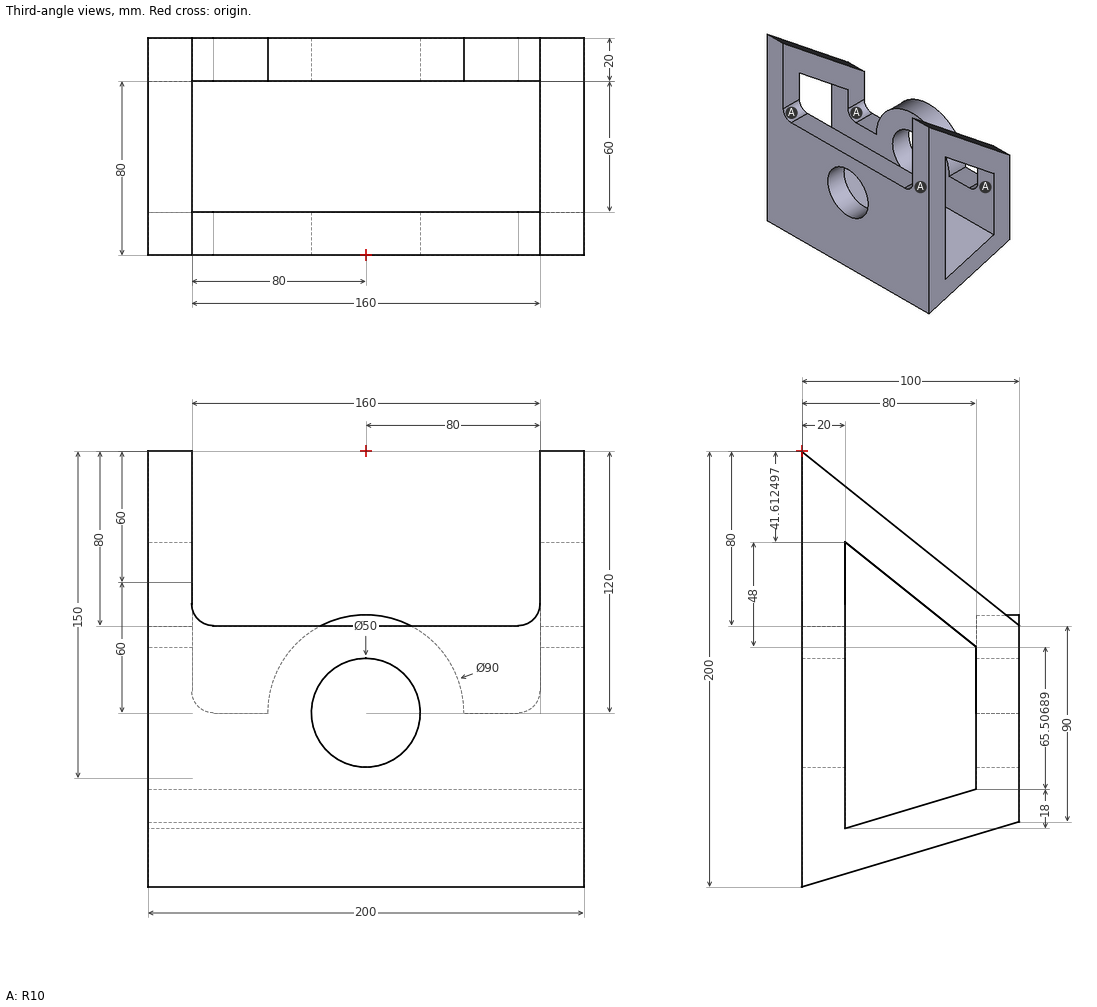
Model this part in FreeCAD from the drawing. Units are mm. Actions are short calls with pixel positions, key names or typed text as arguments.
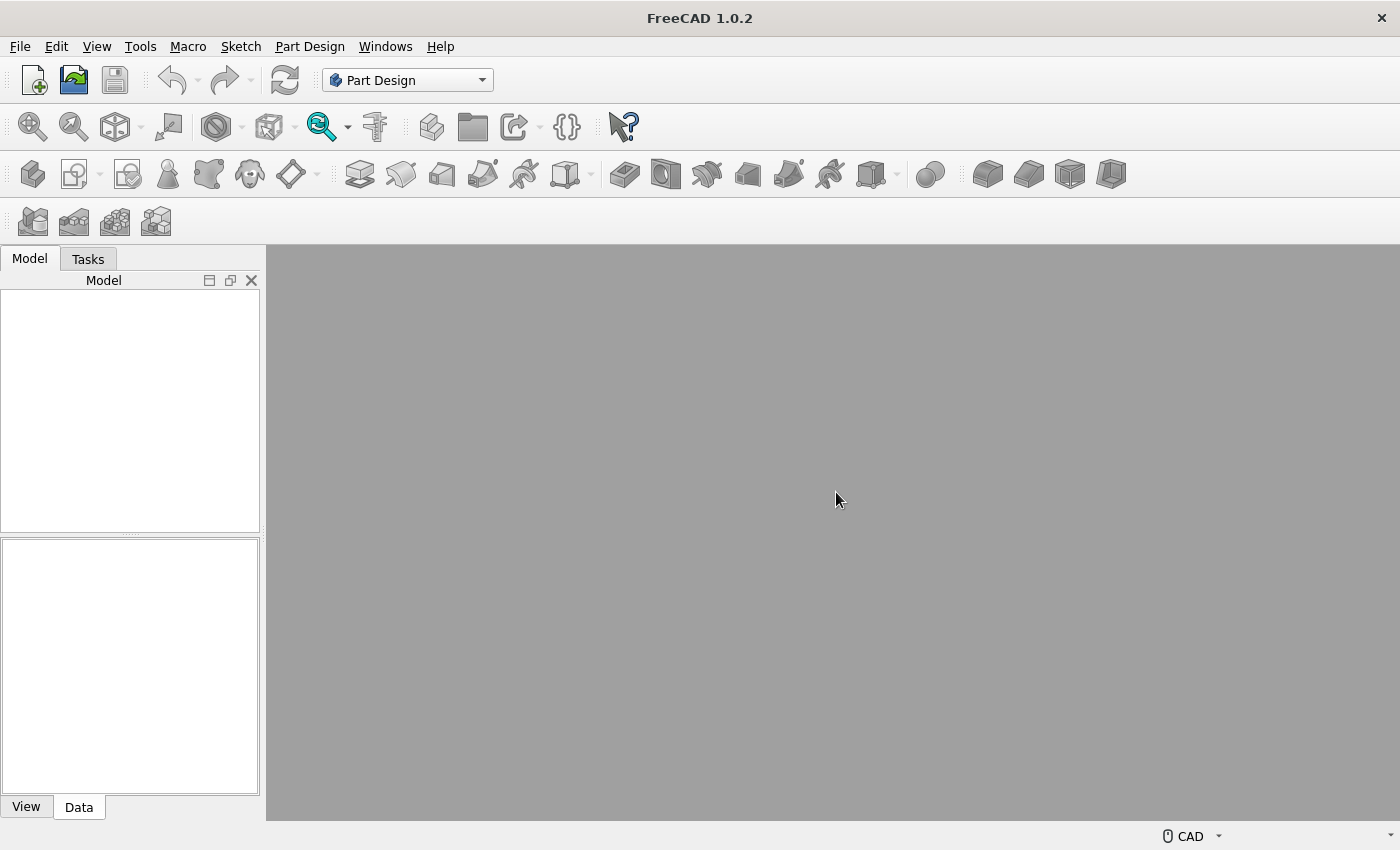
click(33, 80)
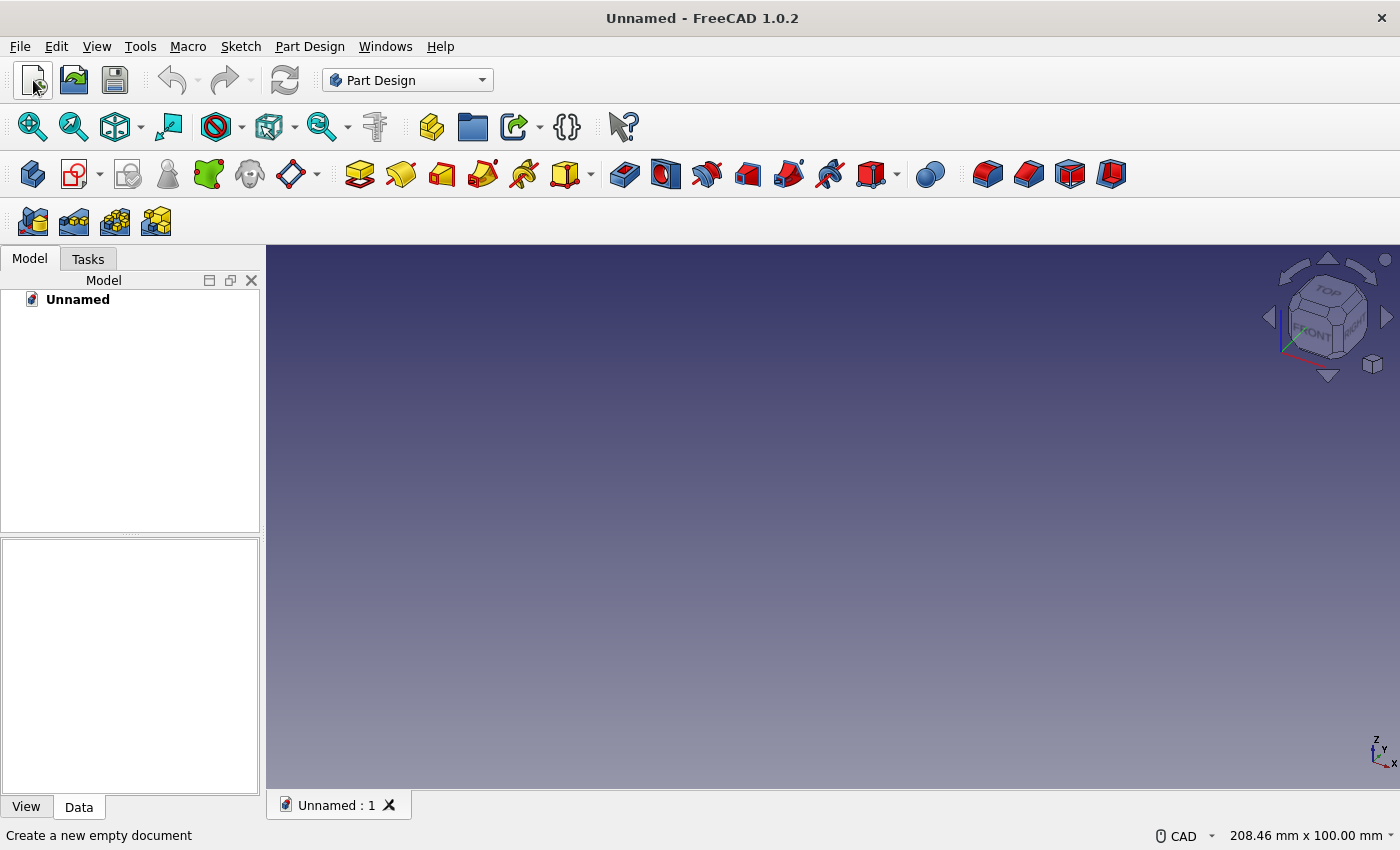
click(74, 174)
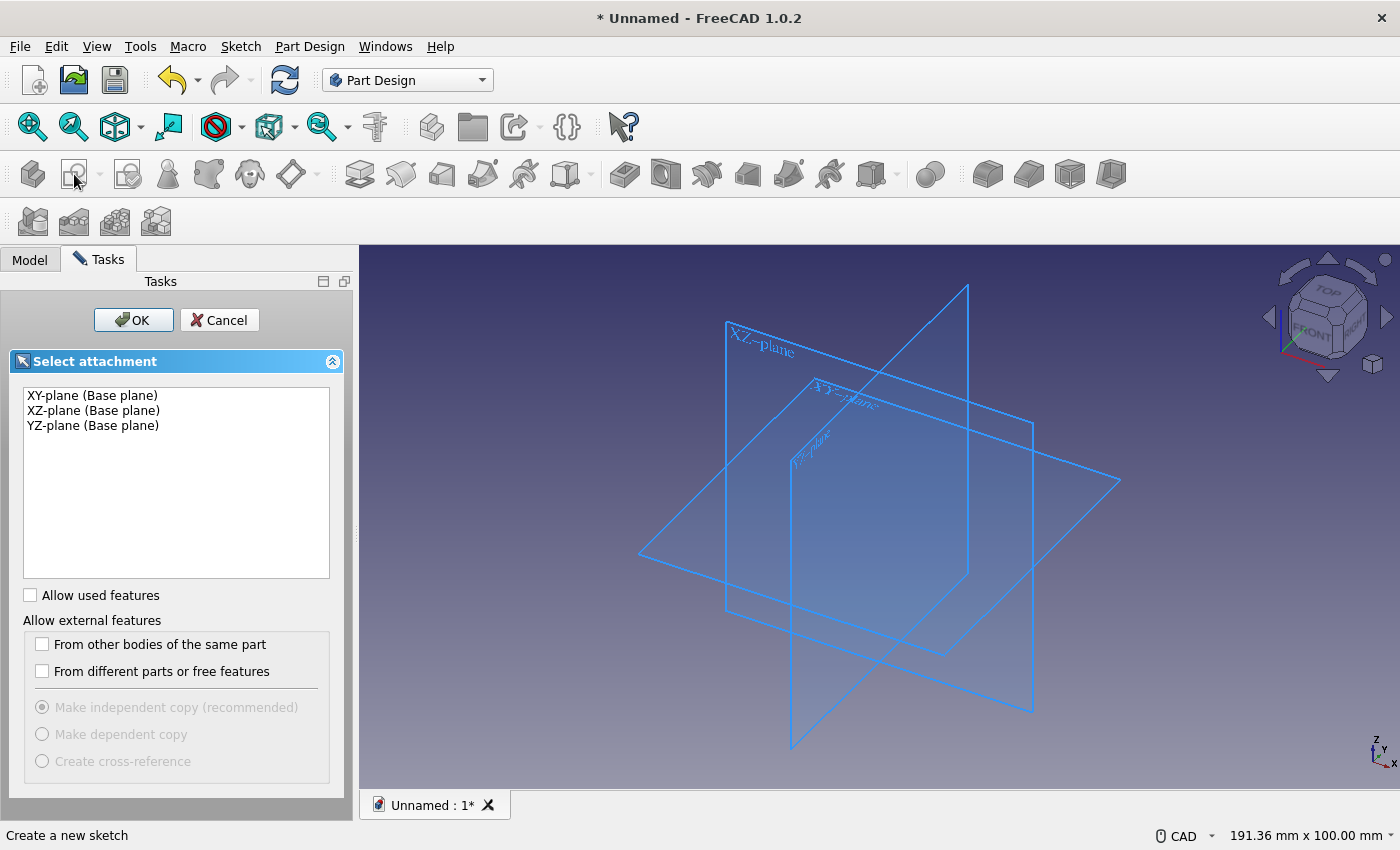
click(84, 426)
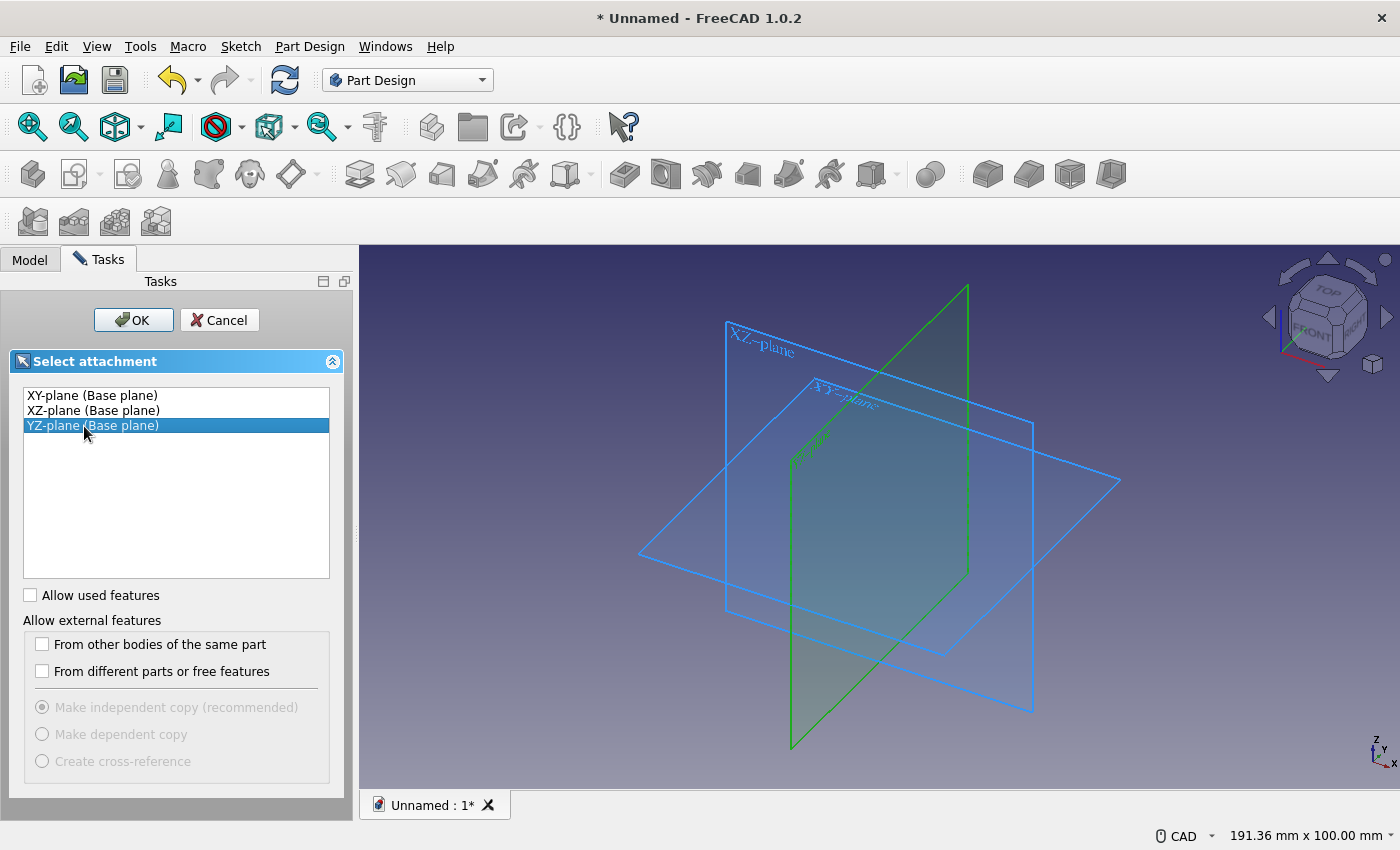
click(134, 320)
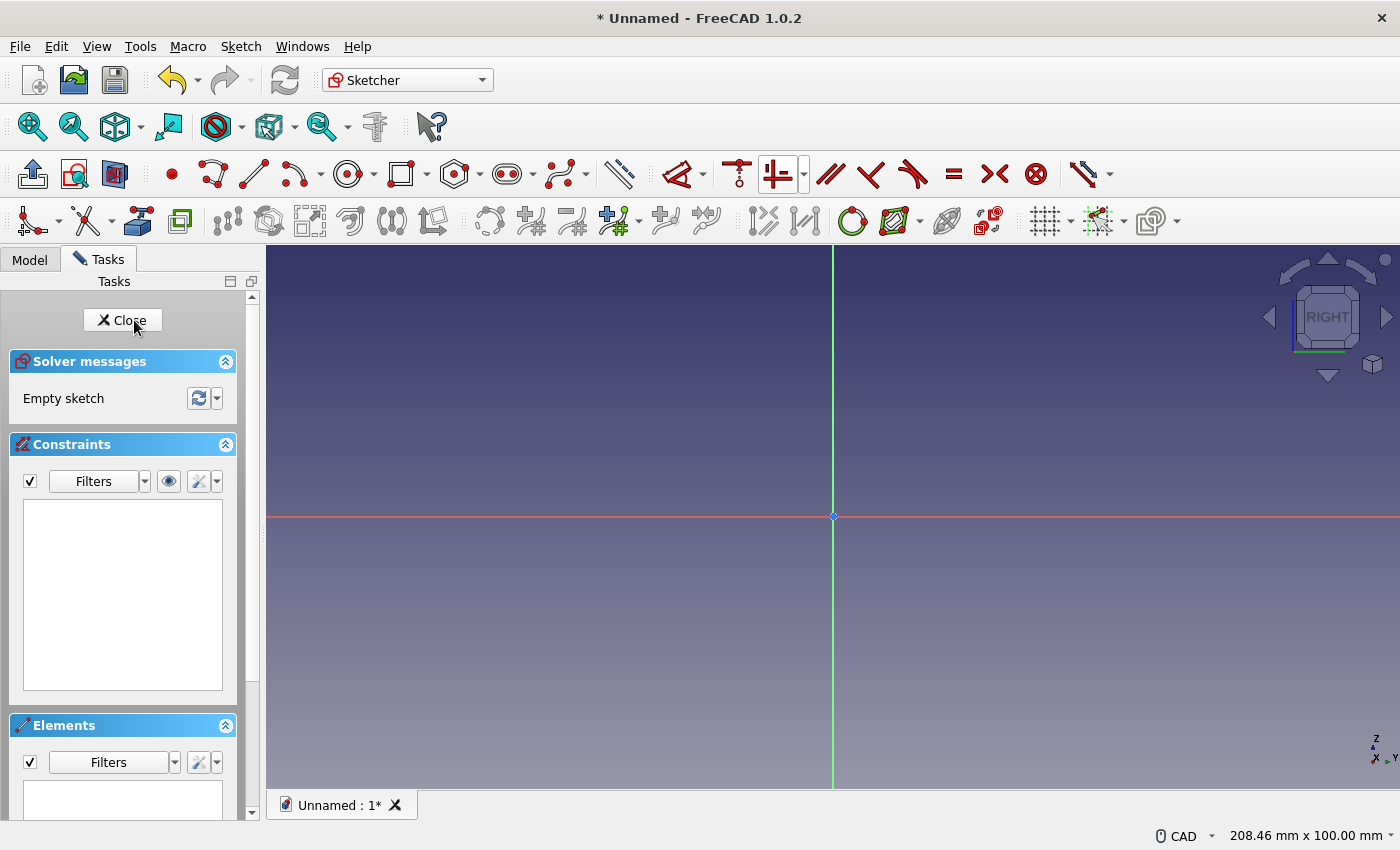
scroll(618, 283, down, 6)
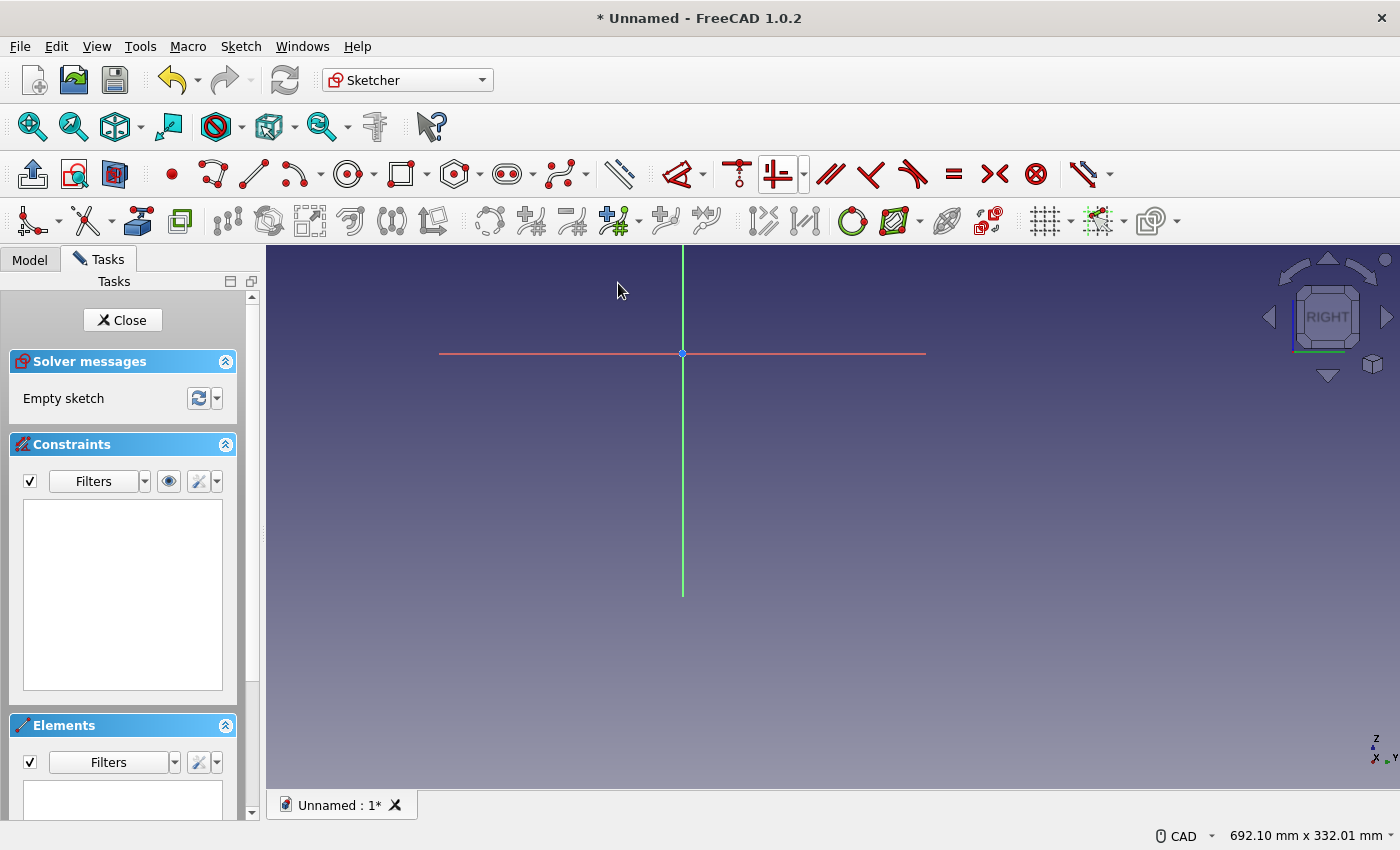
click(213, 174)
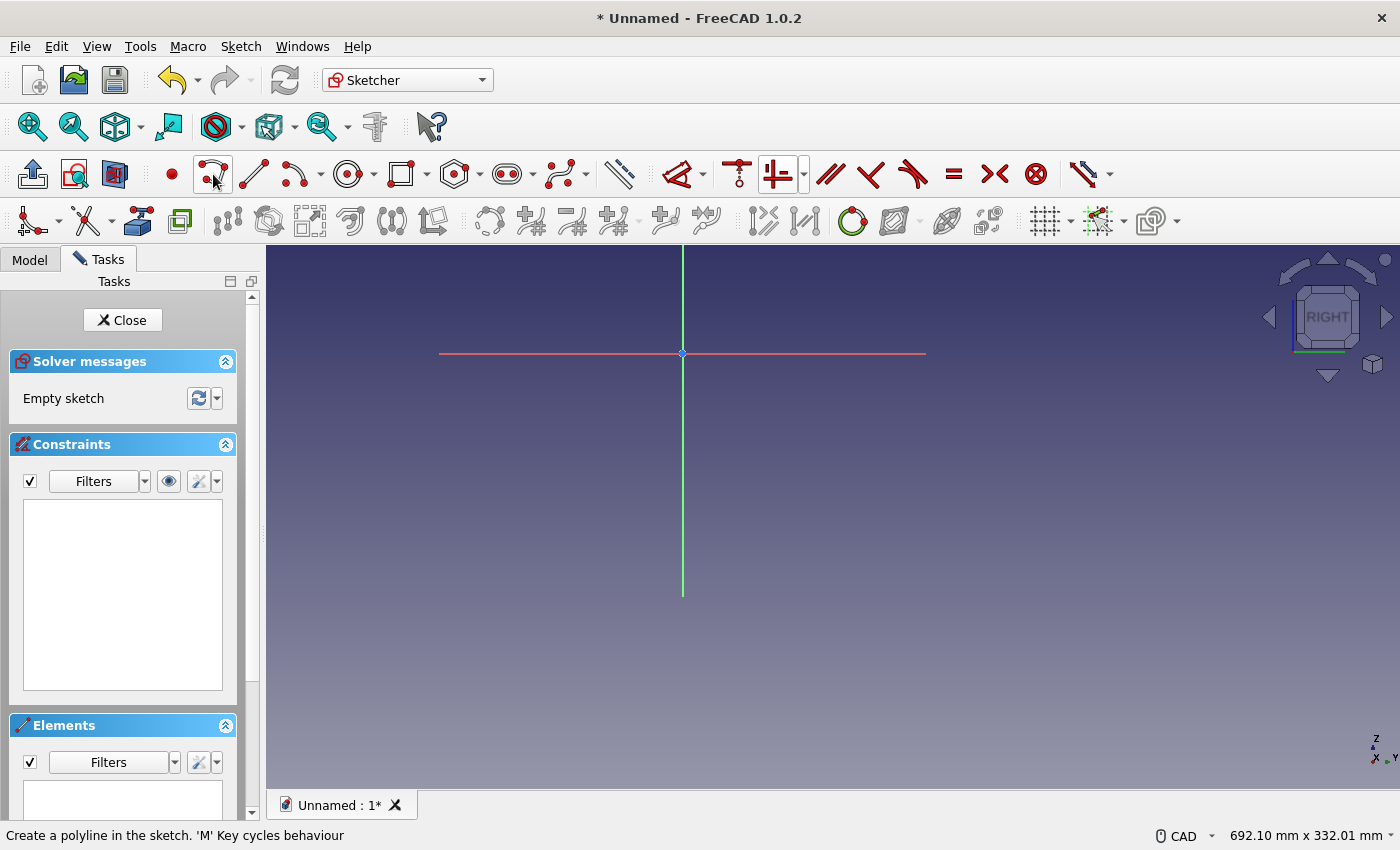
click(683, 354)
click(692, 681)
click(847, 632)
click(847, 485)
click(683, 354)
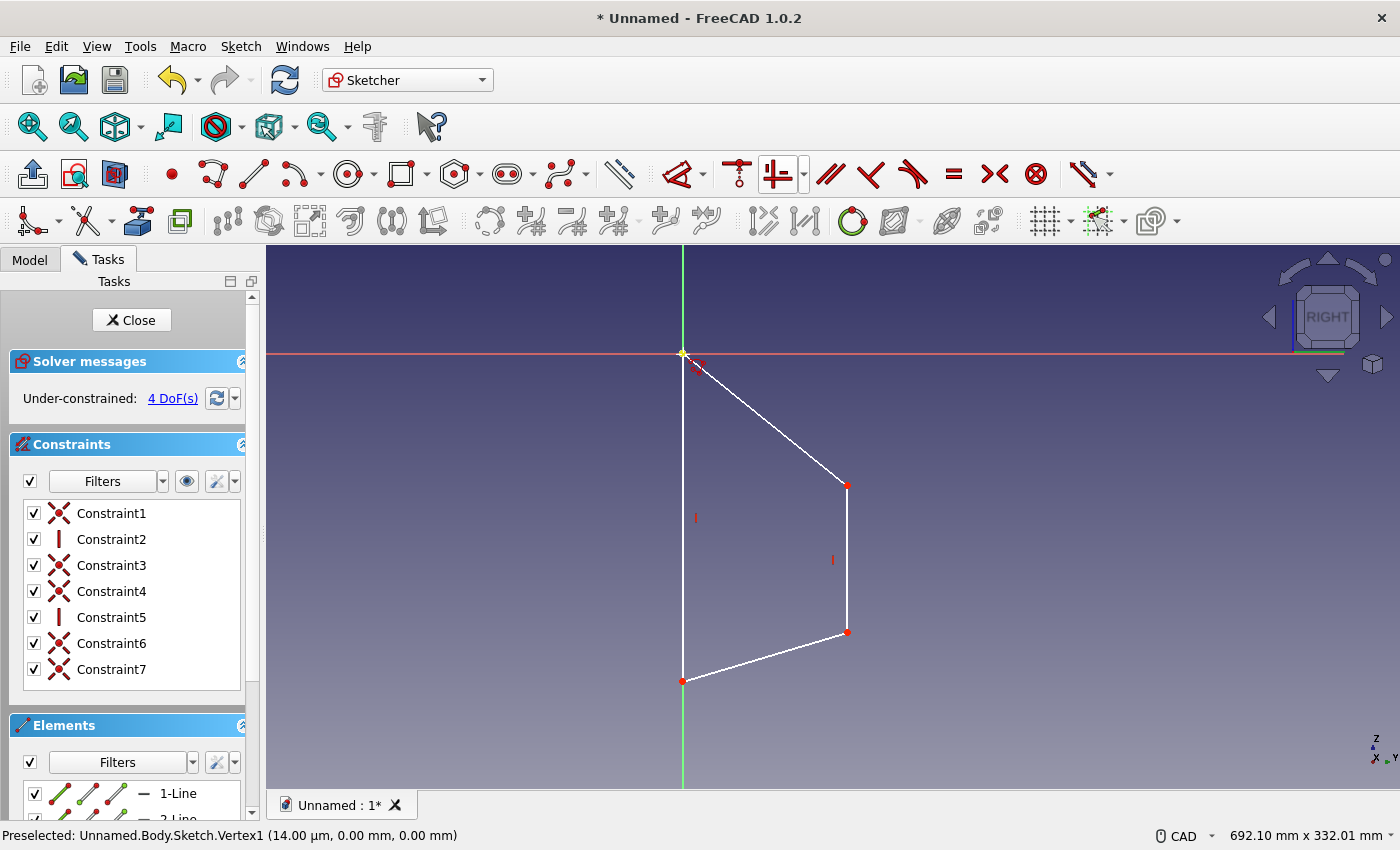
click(716, 422)
click(814, 500)
click(814, 608)
click(716, 637)
click(716, 423)
key(Escape)
key(Escape)